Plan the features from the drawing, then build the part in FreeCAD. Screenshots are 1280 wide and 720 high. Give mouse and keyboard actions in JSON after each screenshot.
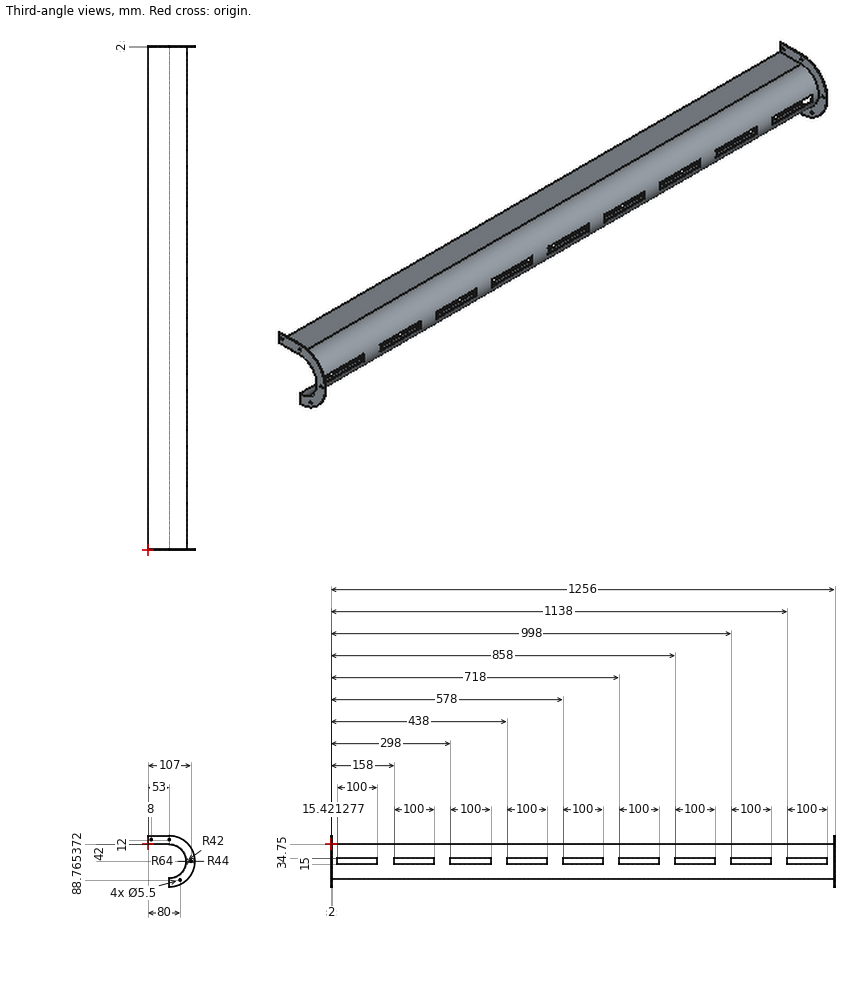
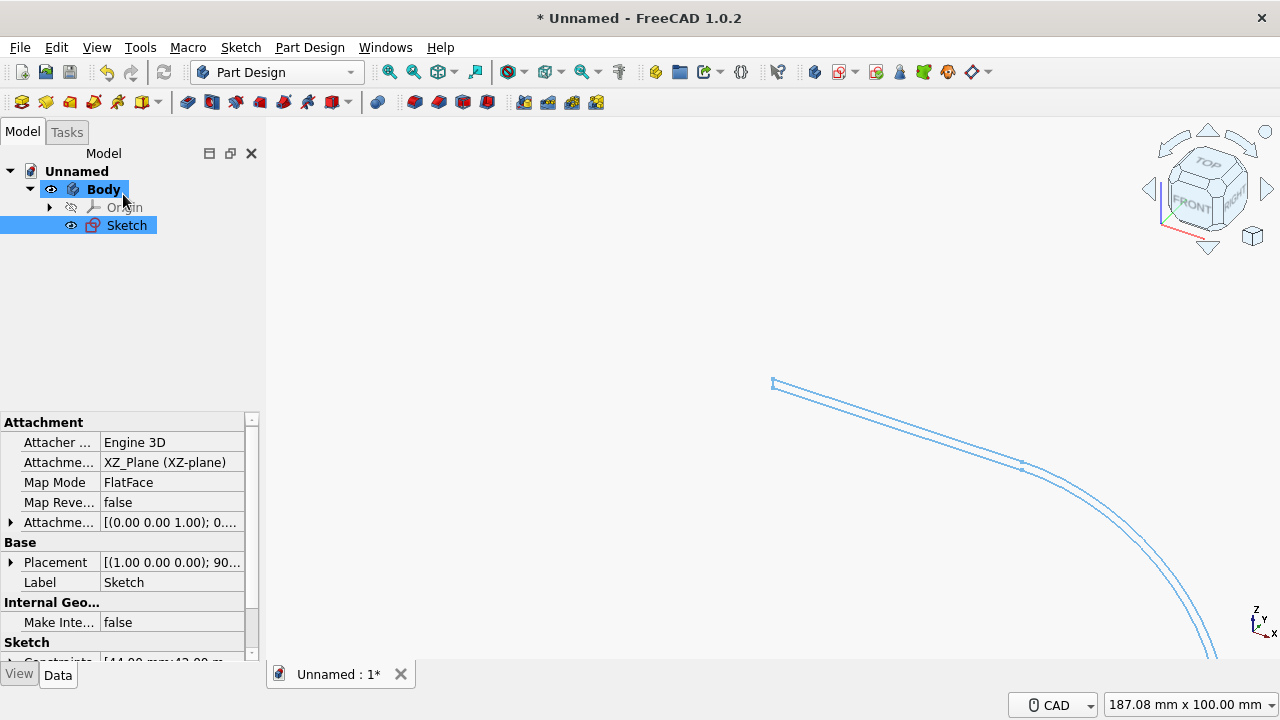
{"action": "left_click", "coordinate": [22, 102]}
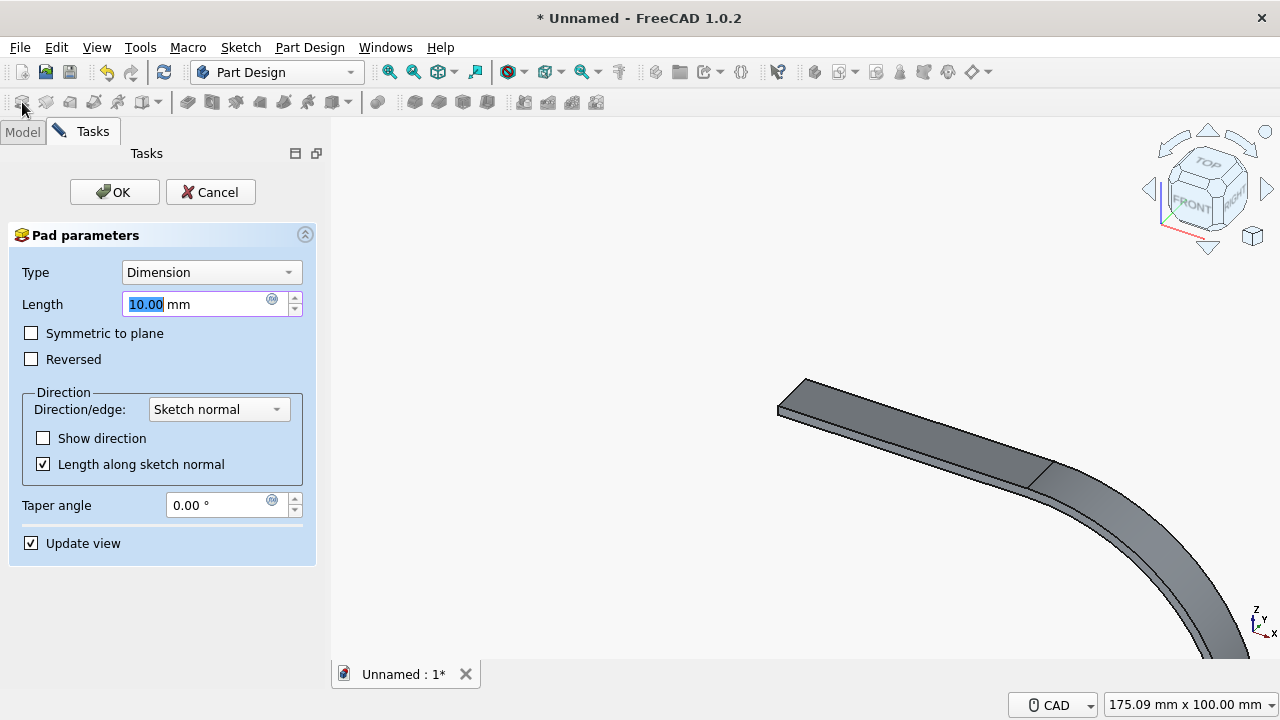
{"action": "type", "text": "1256"}
{"action": "key", "text": "Tab"}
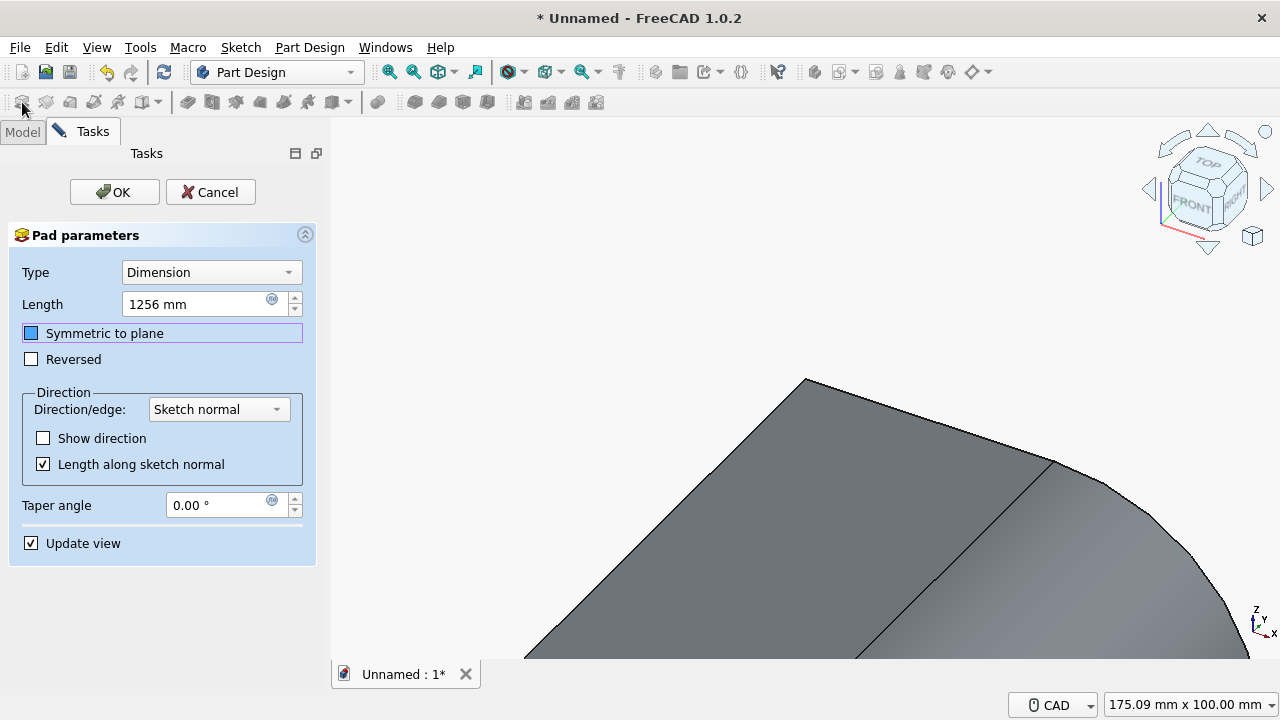
{"action": "left_click", "coordinate": [30, 359]}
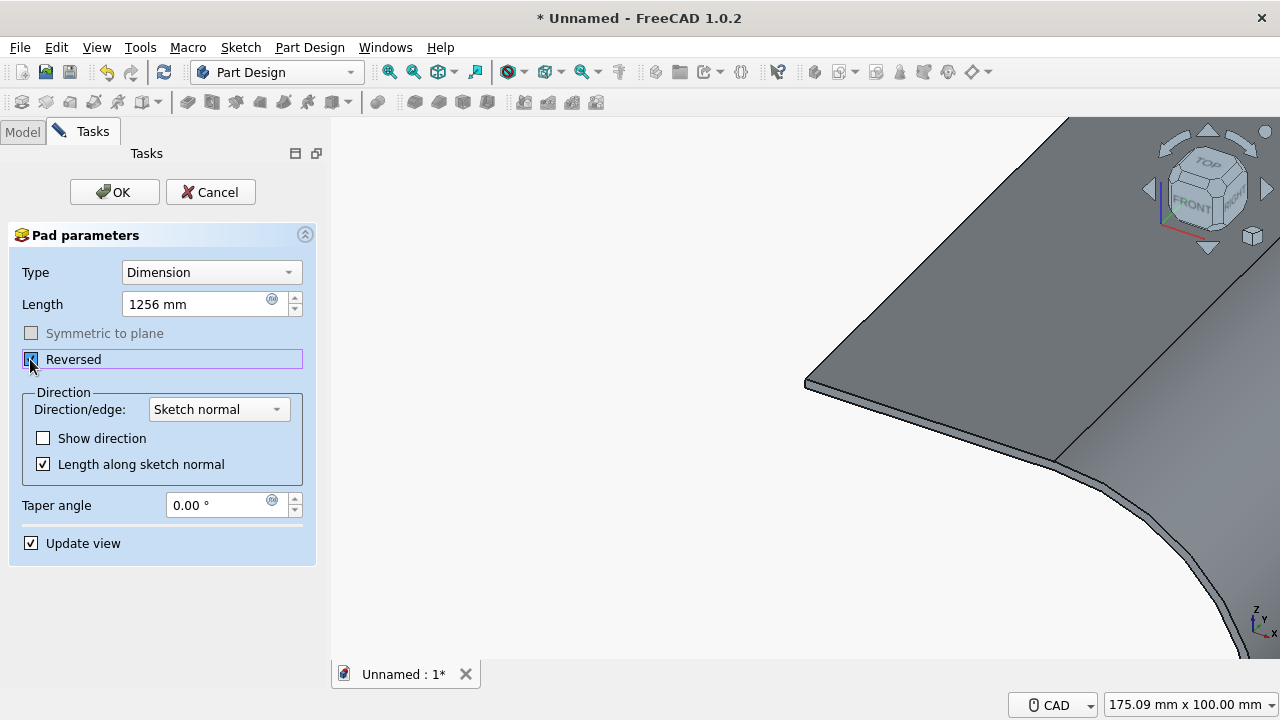
{"action": "left_click", "coordinate": [115, 192]}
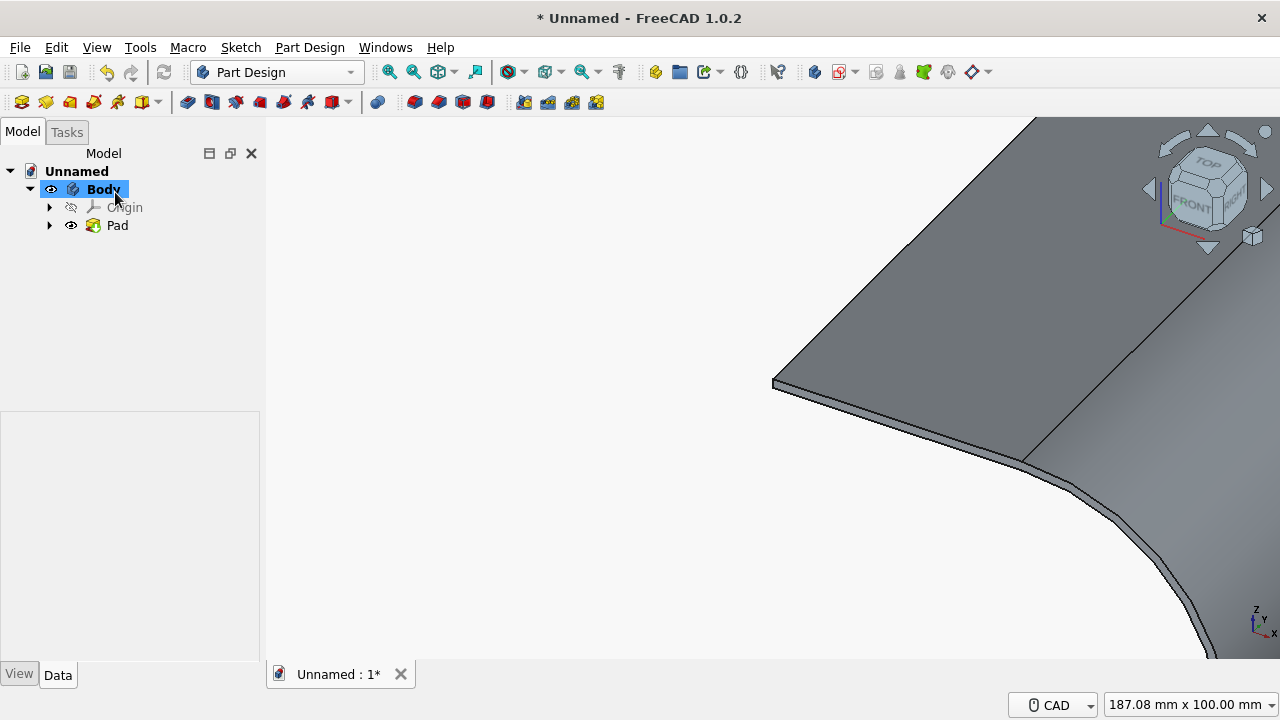
{"action": "left_click", "coordinate": [390, 72]}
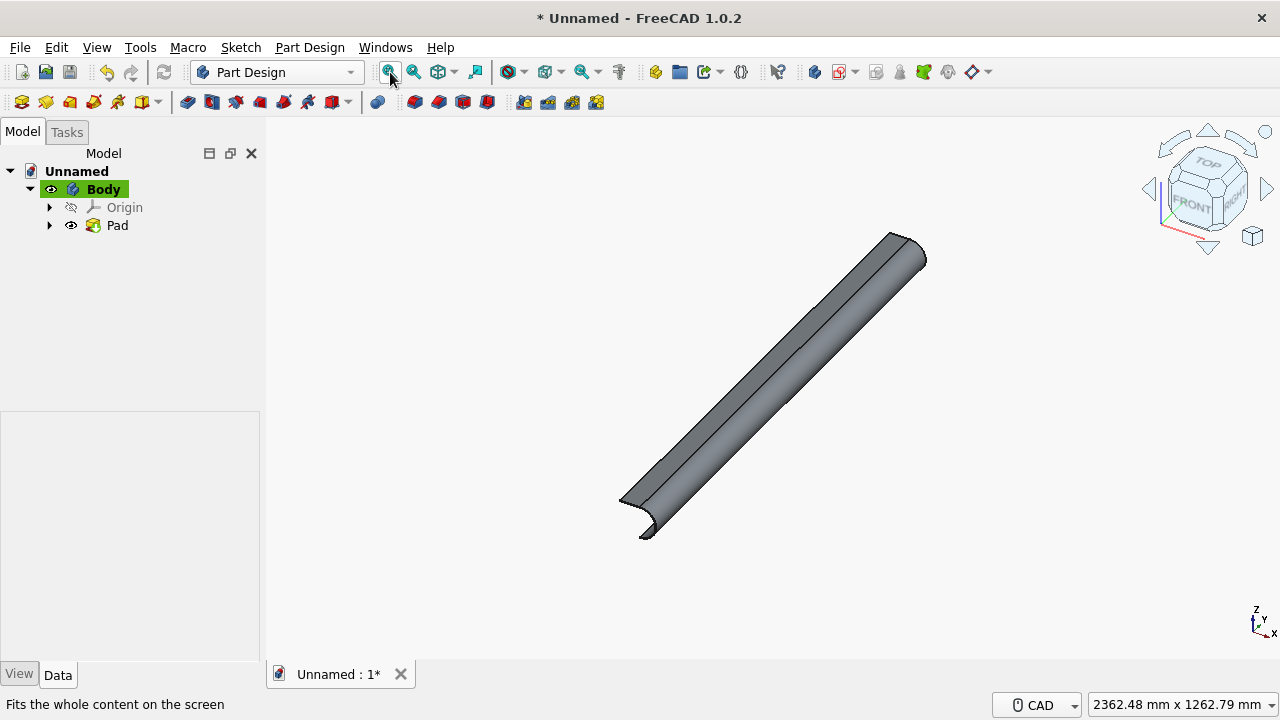
{"action": "left_click", "coordinate": [50, 207]}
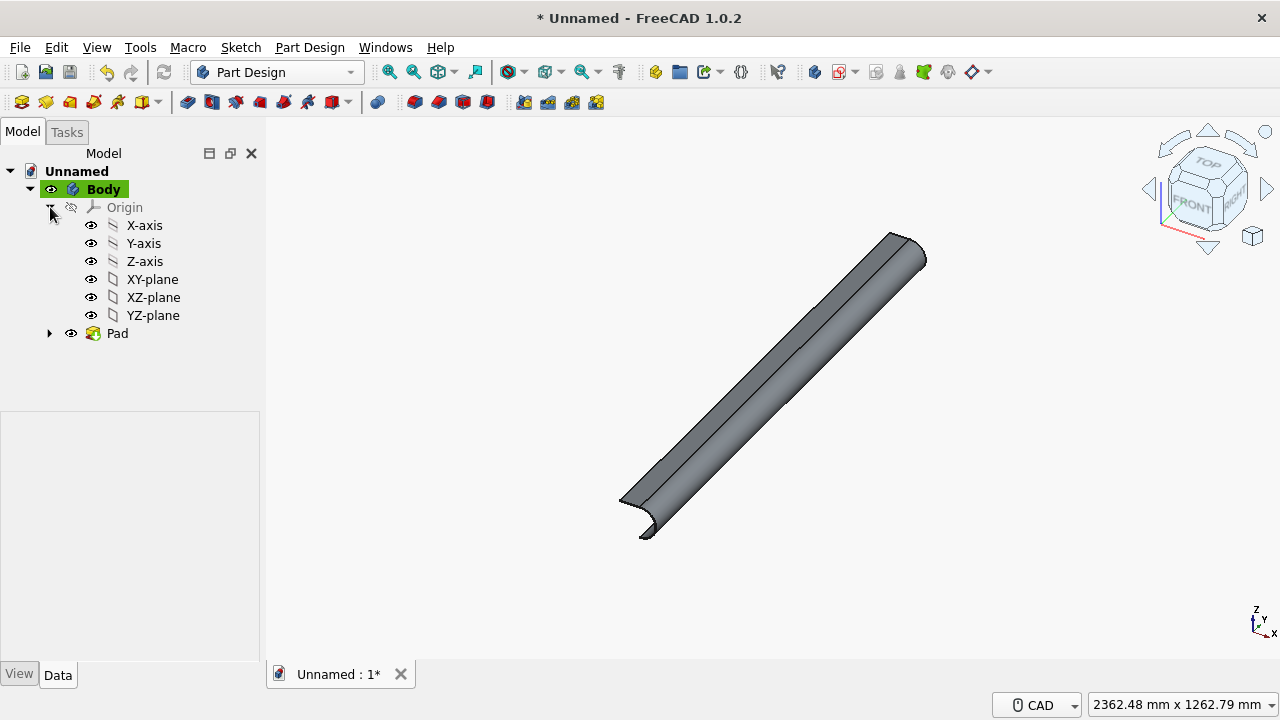
{"action": "left_click", "coordinate": [136, 297]}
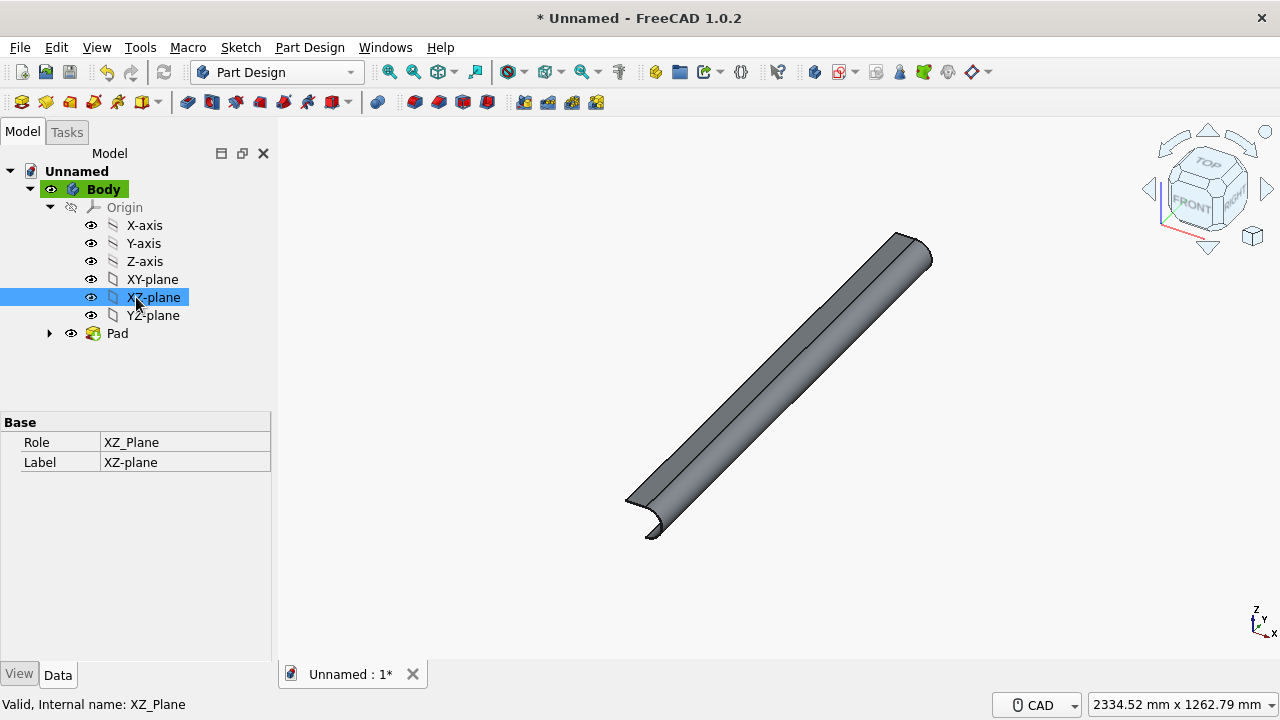
{"action": "left_click", "coordinate": [972, 72]}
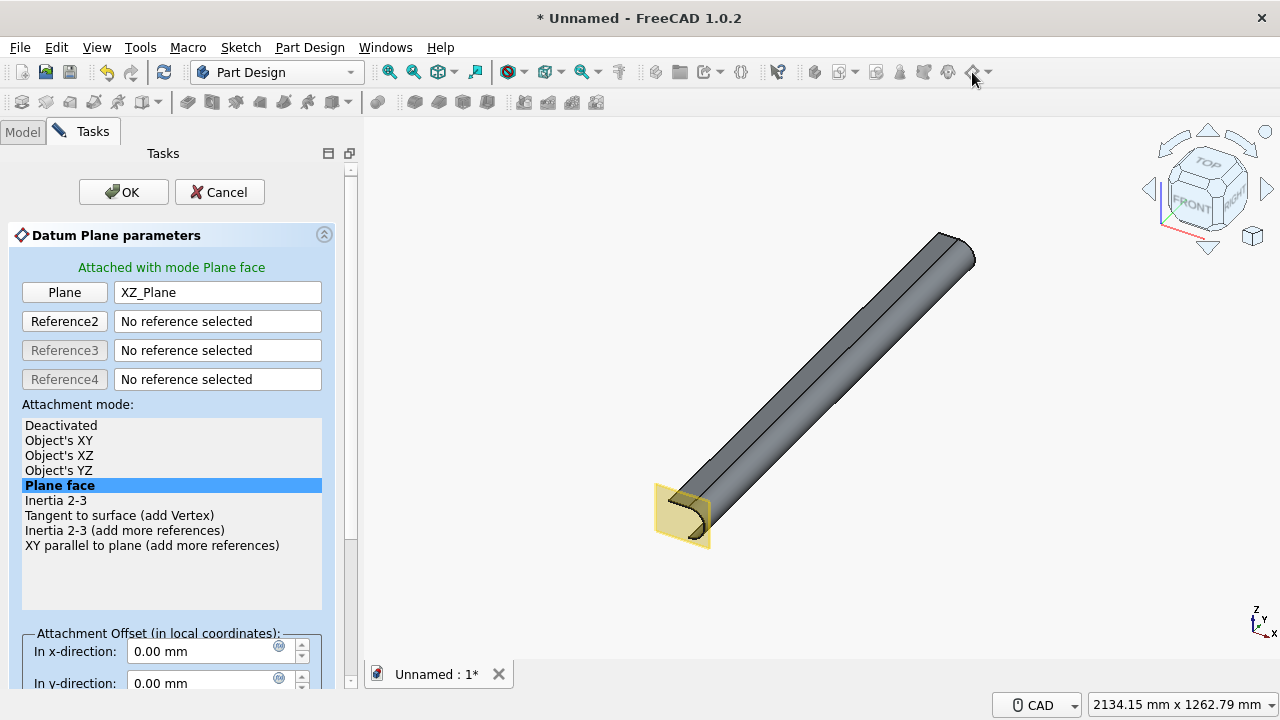
{"action": "scroll", "coordinate": [351, 426], "scroll_direction": "down", "scroll_amount": 2}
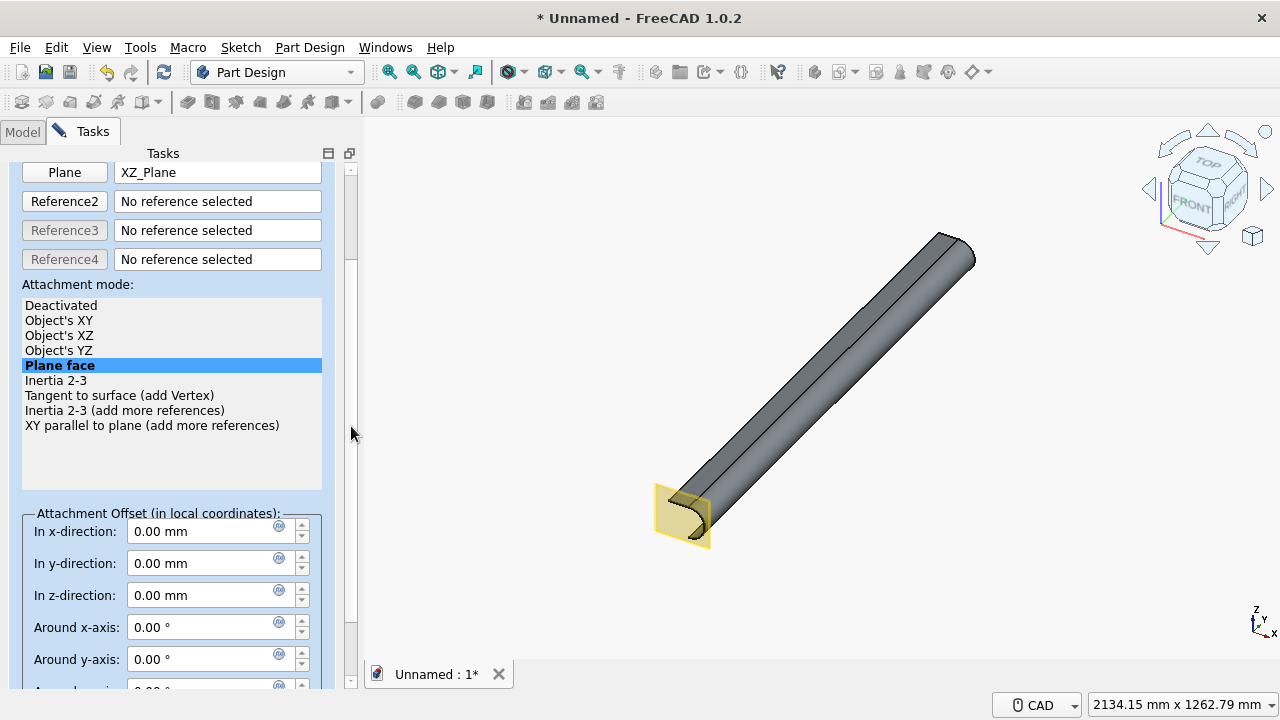
{"action": "triple_click", "coordinate": [210, 595]}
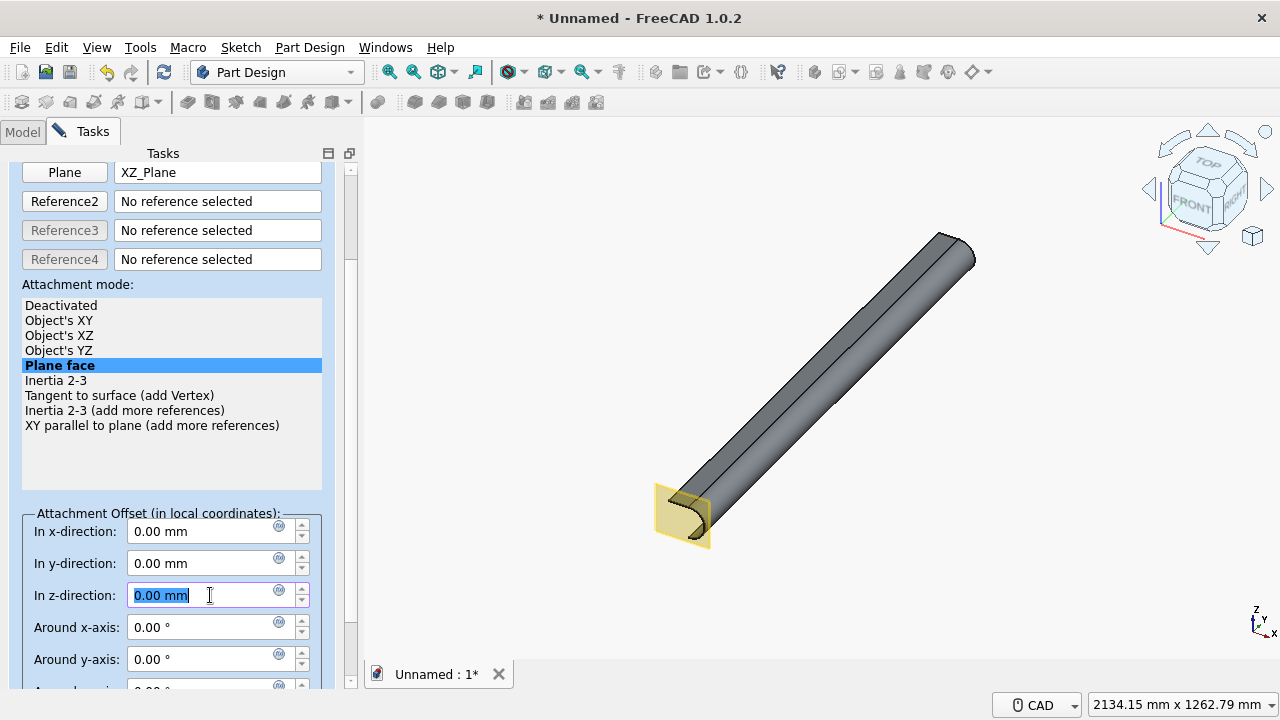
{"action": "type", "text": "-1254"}
{"action": "key", "text": "Tab"}